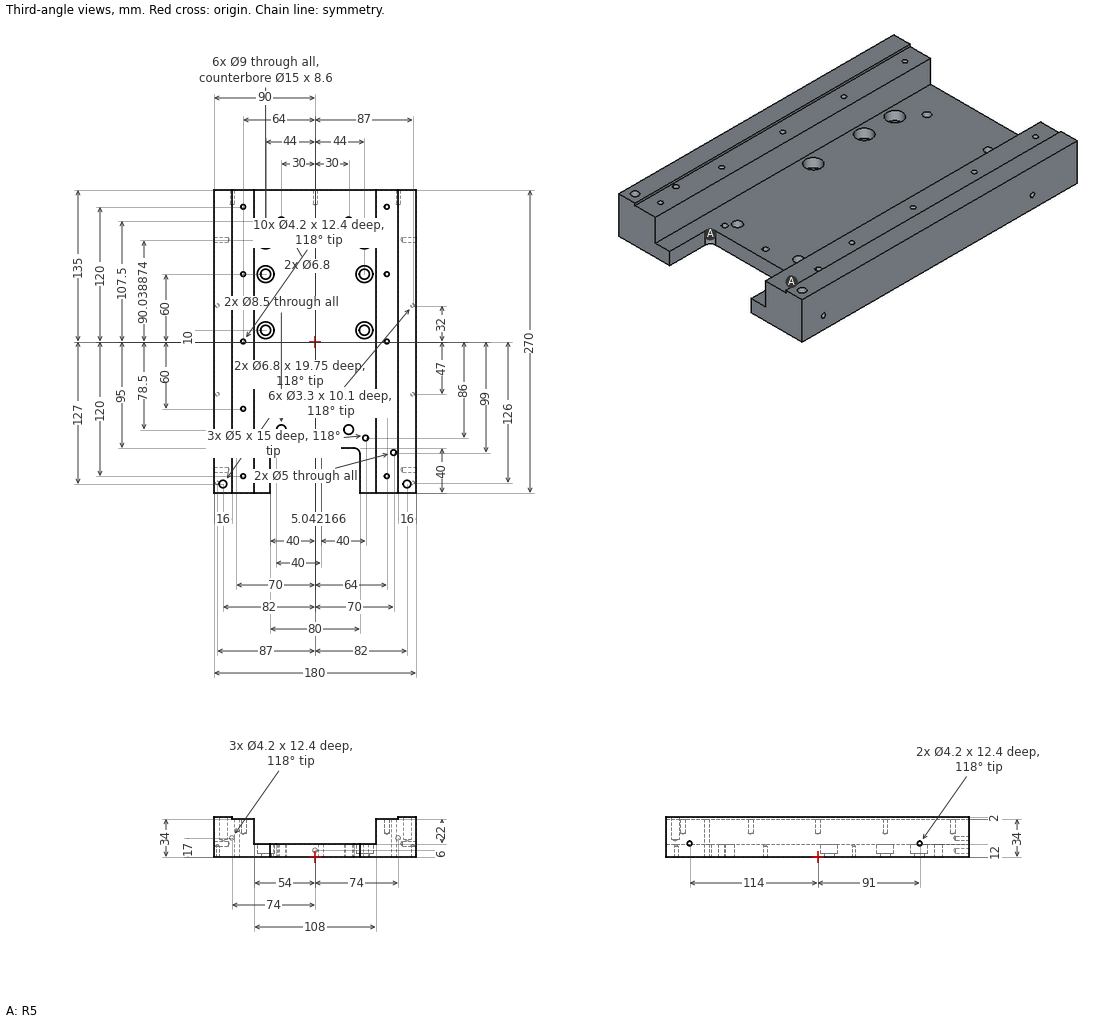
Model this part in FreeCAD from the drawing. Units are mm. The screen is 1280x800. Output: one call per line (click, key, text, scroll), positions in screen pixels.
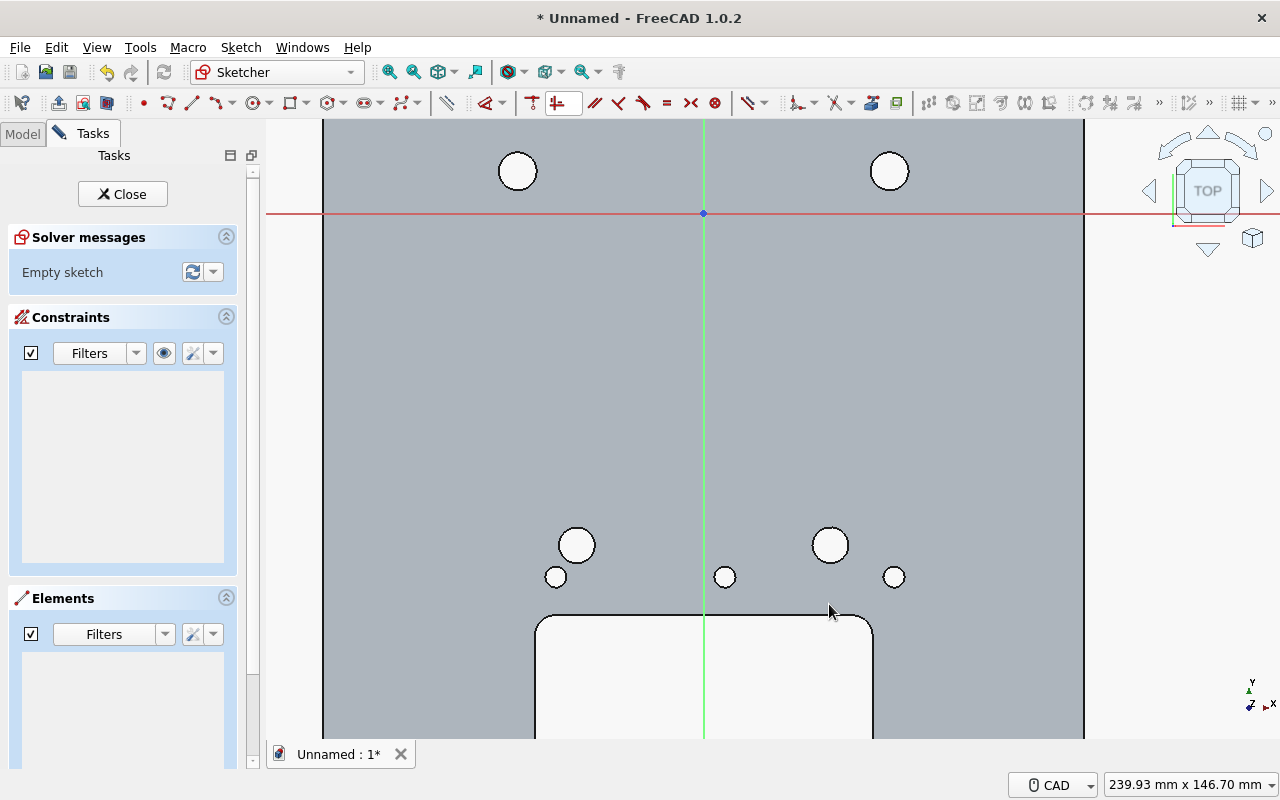
key(g)
key(c)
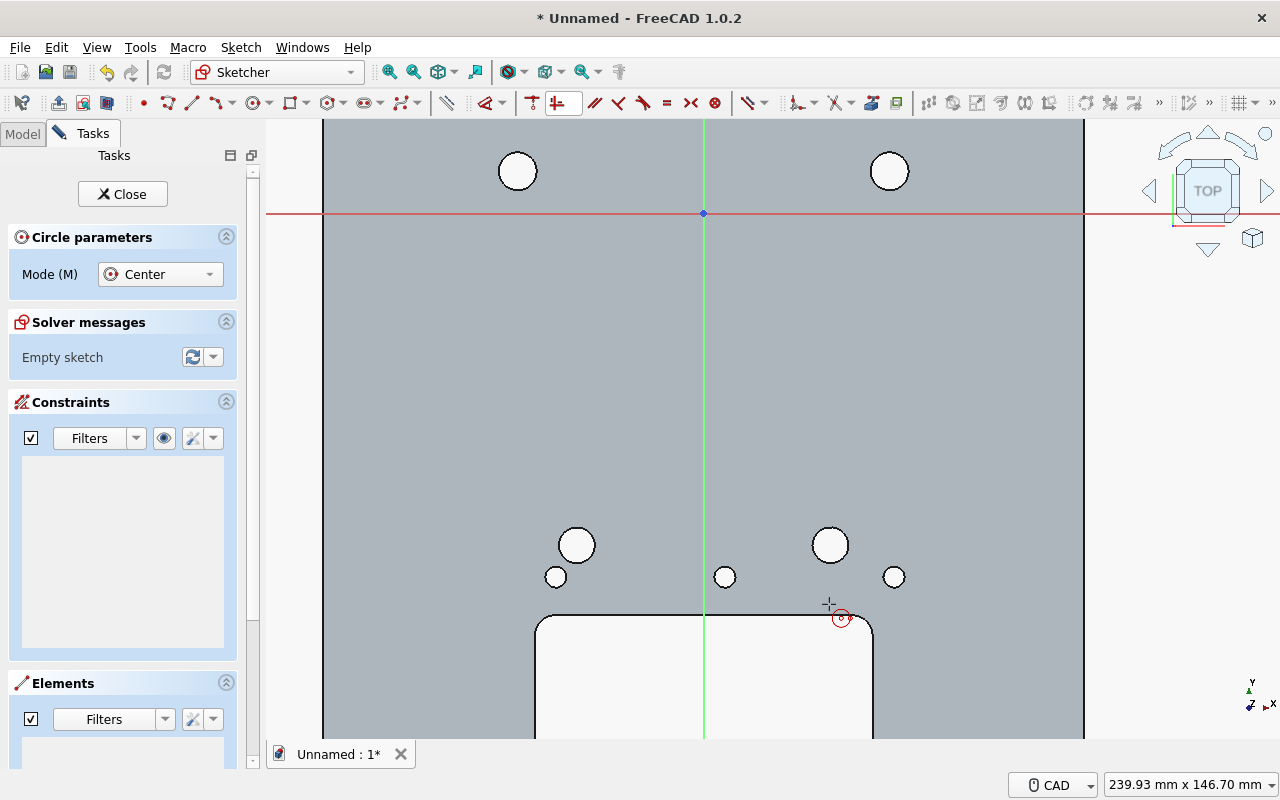
scroll(1000, 632, up, 4)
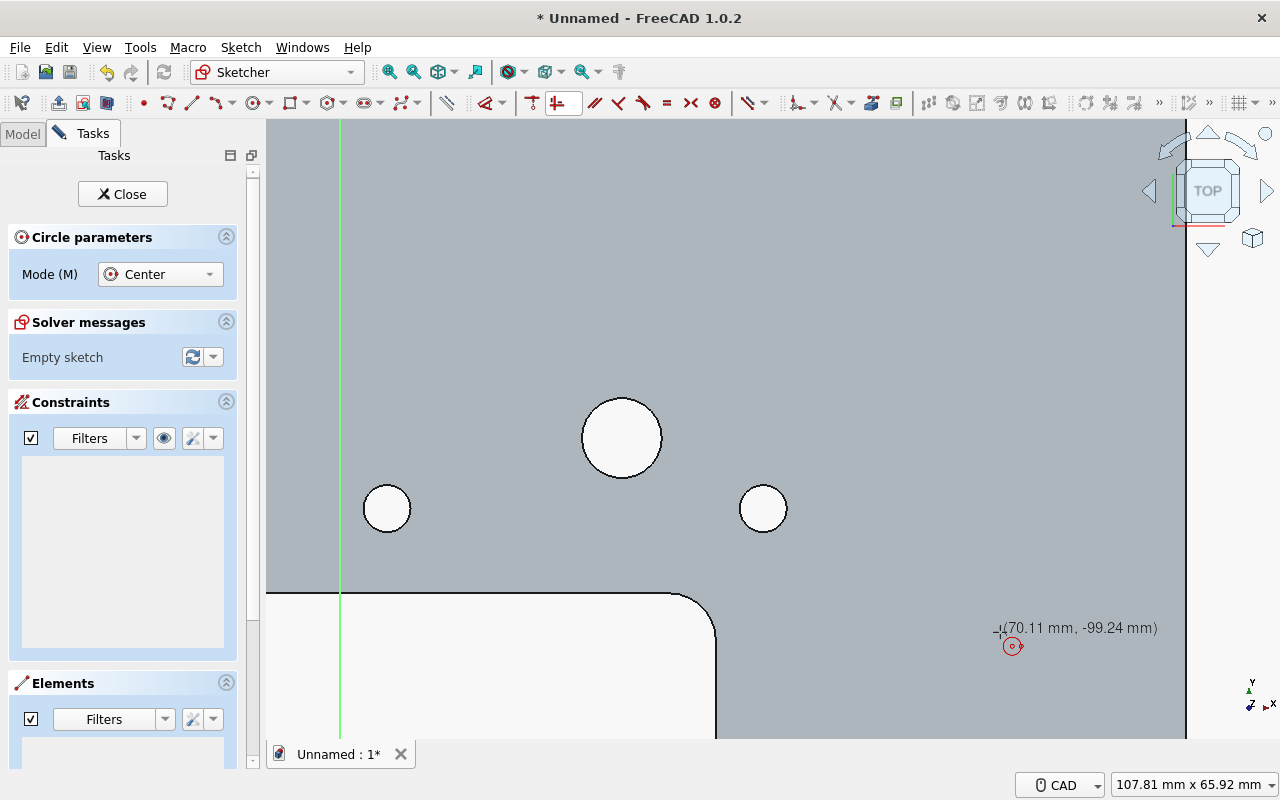
click(998, 631)
move(1015, 614)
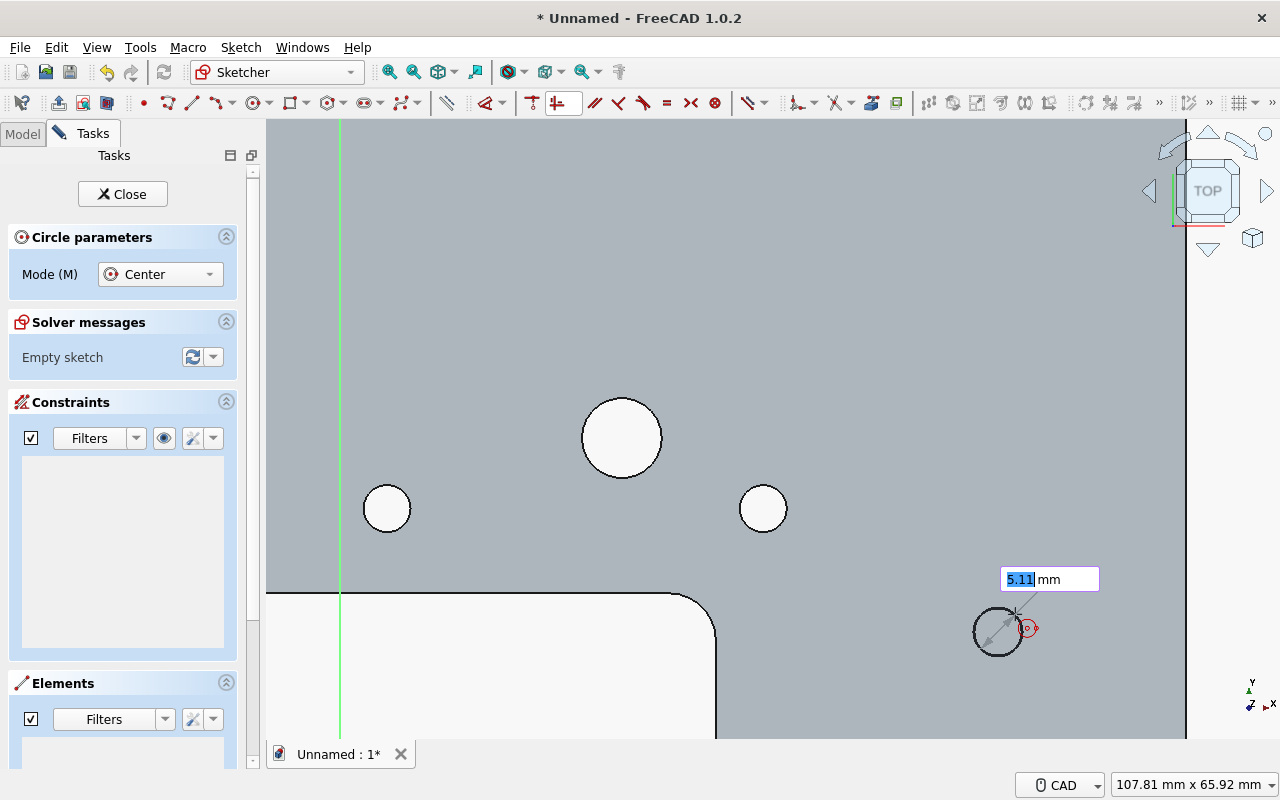
text(5)
key(Return)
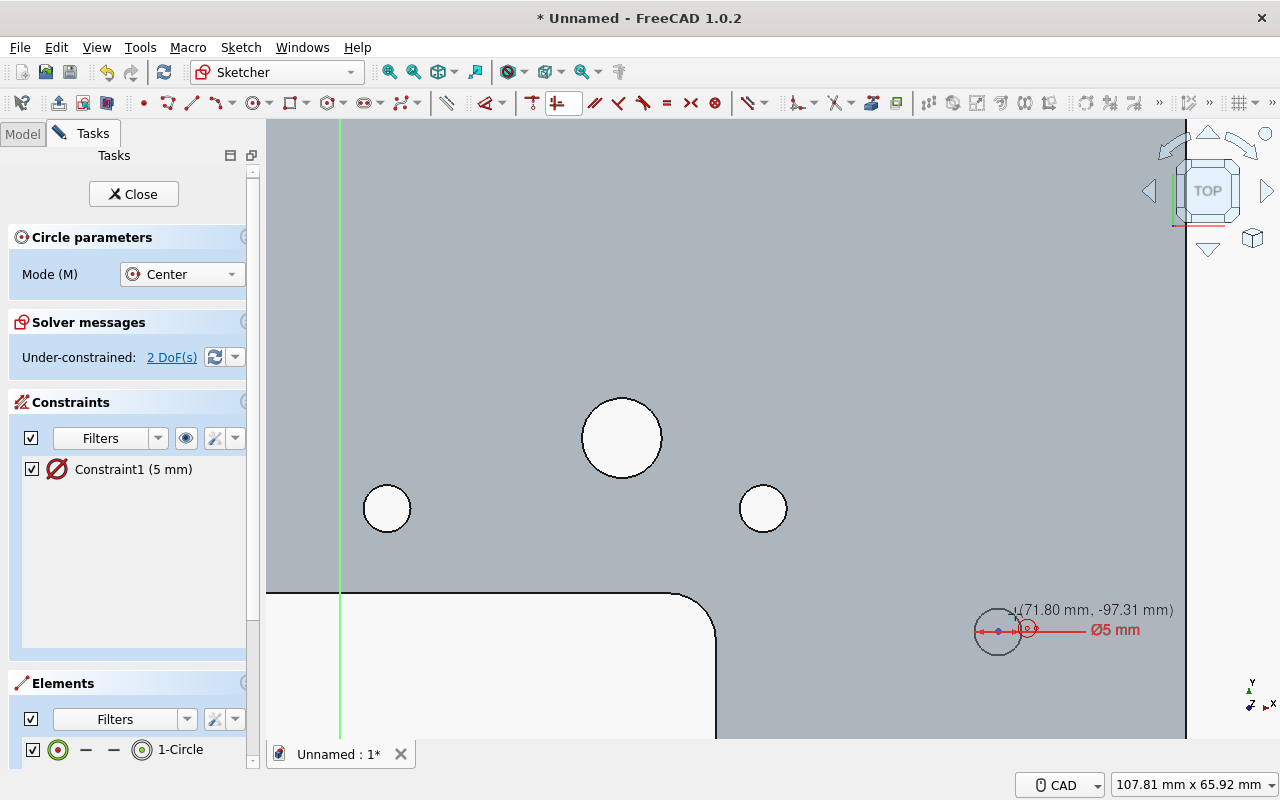
scroll(1002, 635, down, 4)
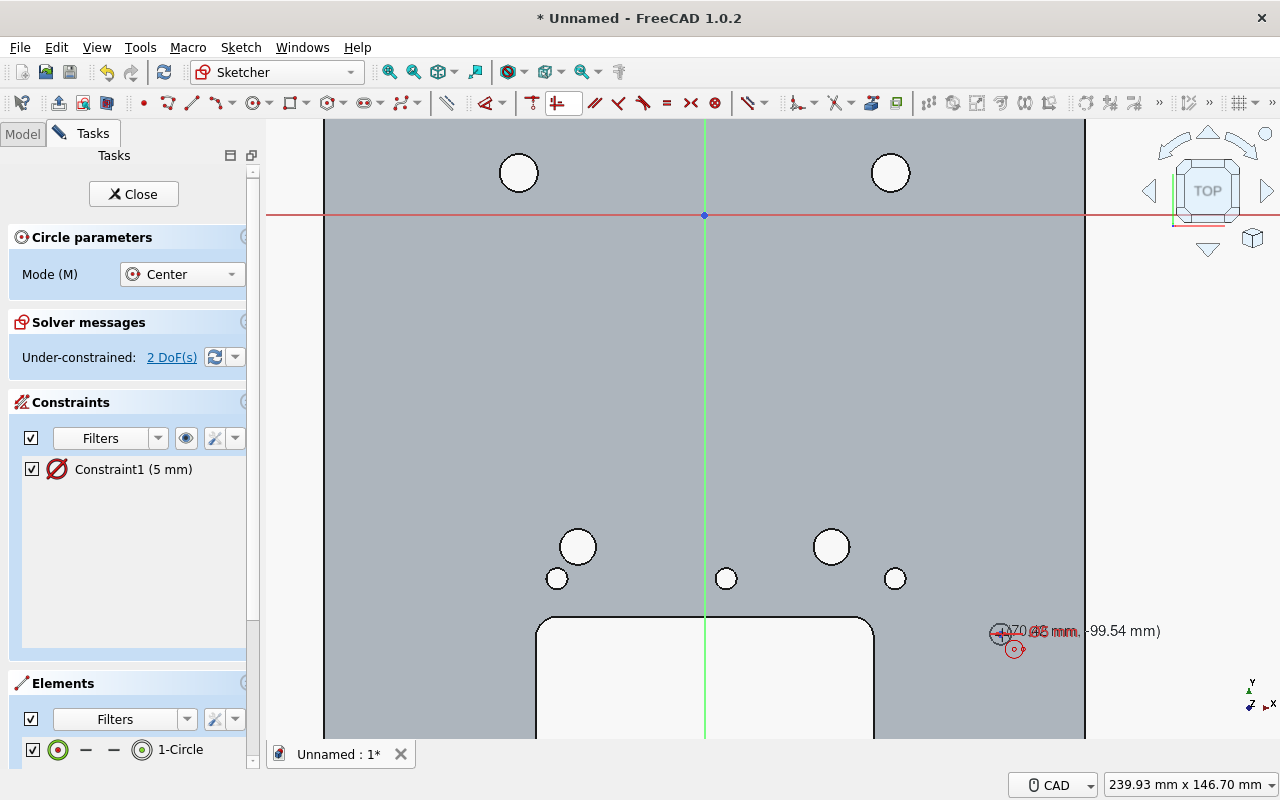
scroll(409, 634, up, 4)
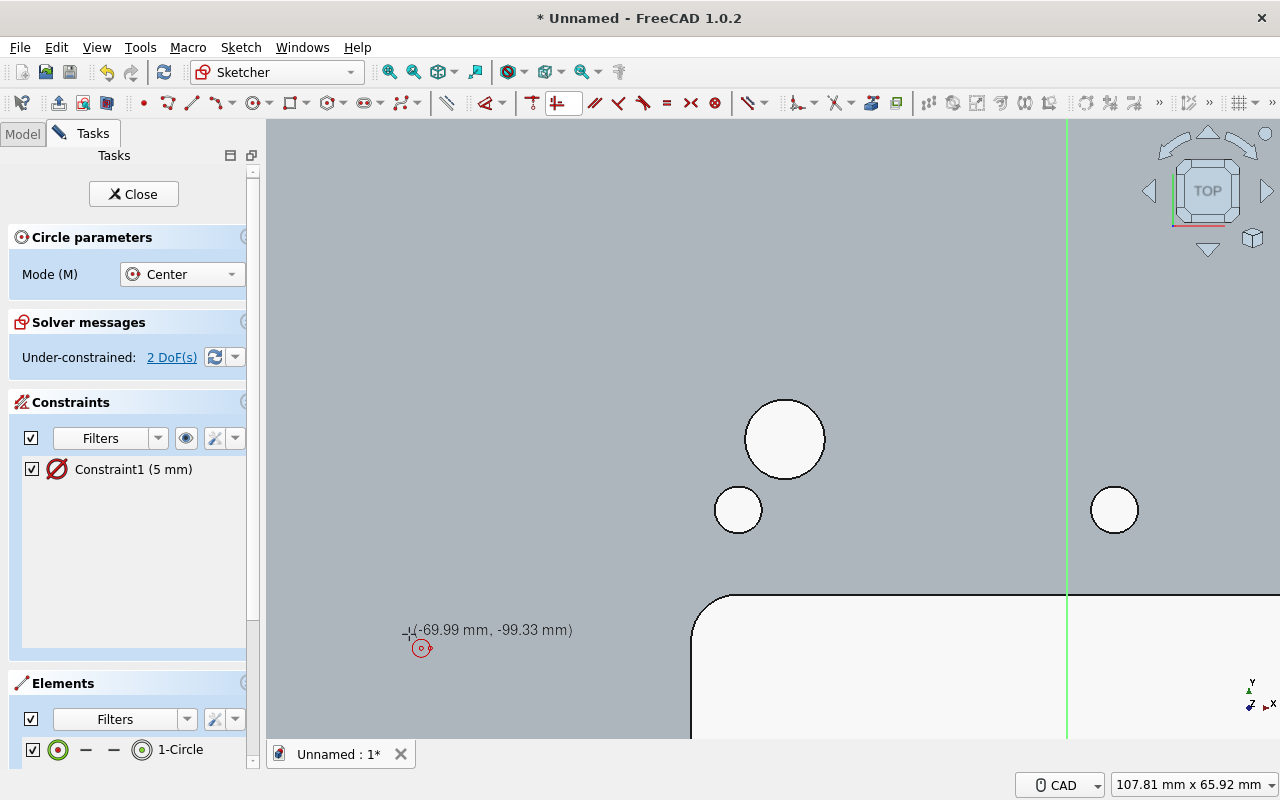
click(409, 632)
move(425, 616)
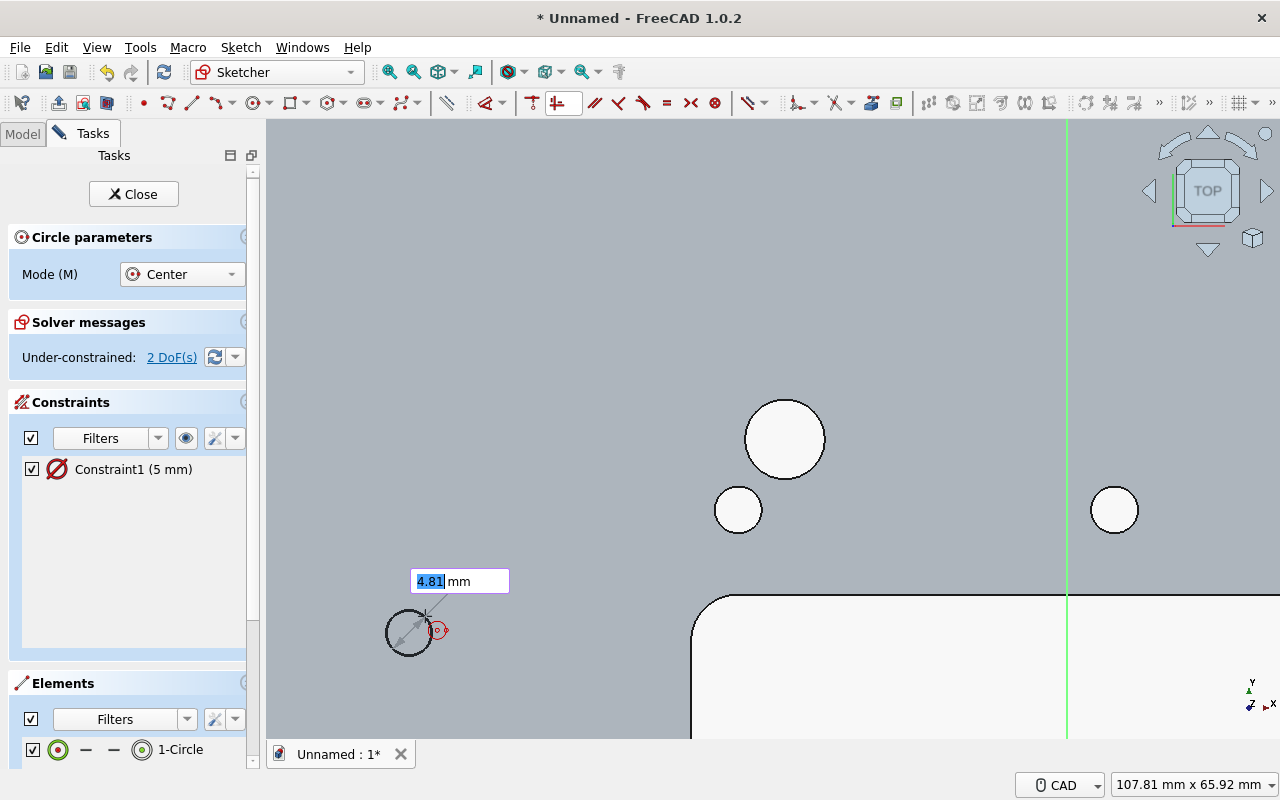
text(5)
key(Return)
key(Escape)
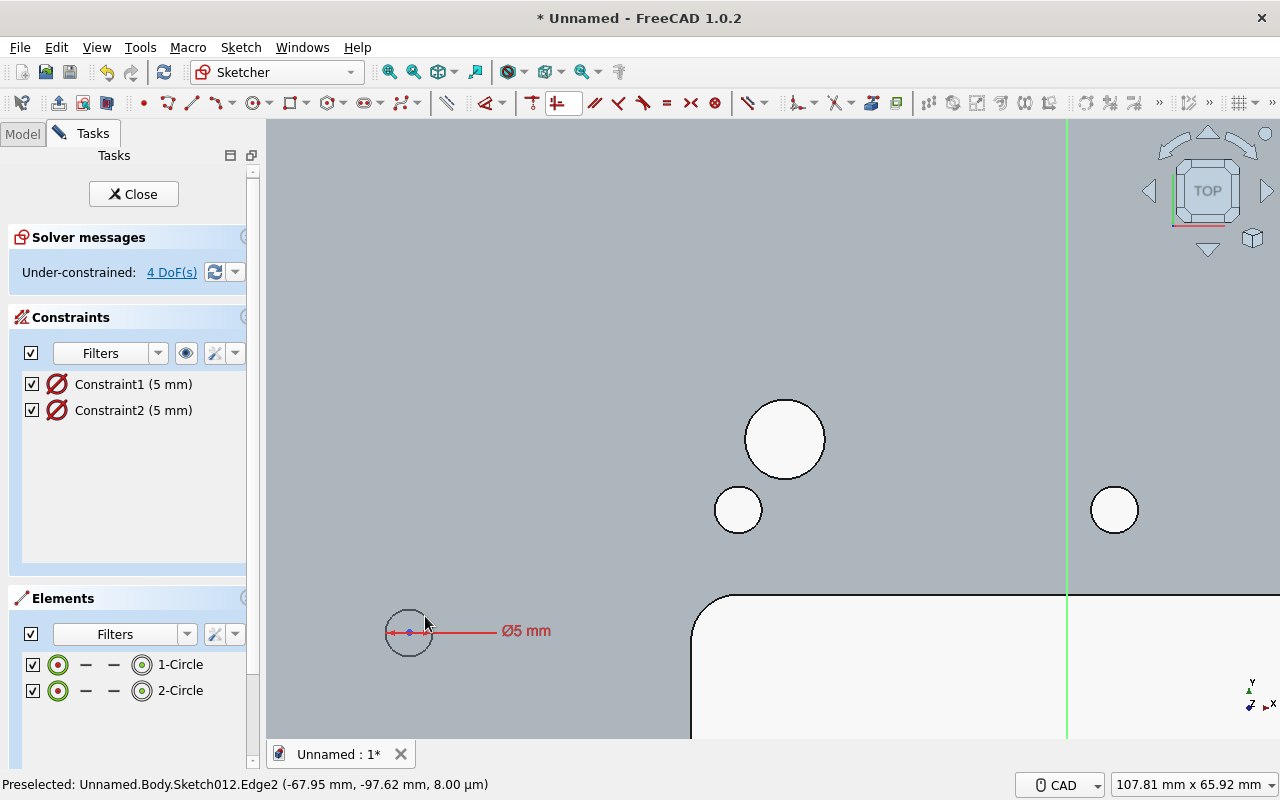
scroll(409, 634, down, 4)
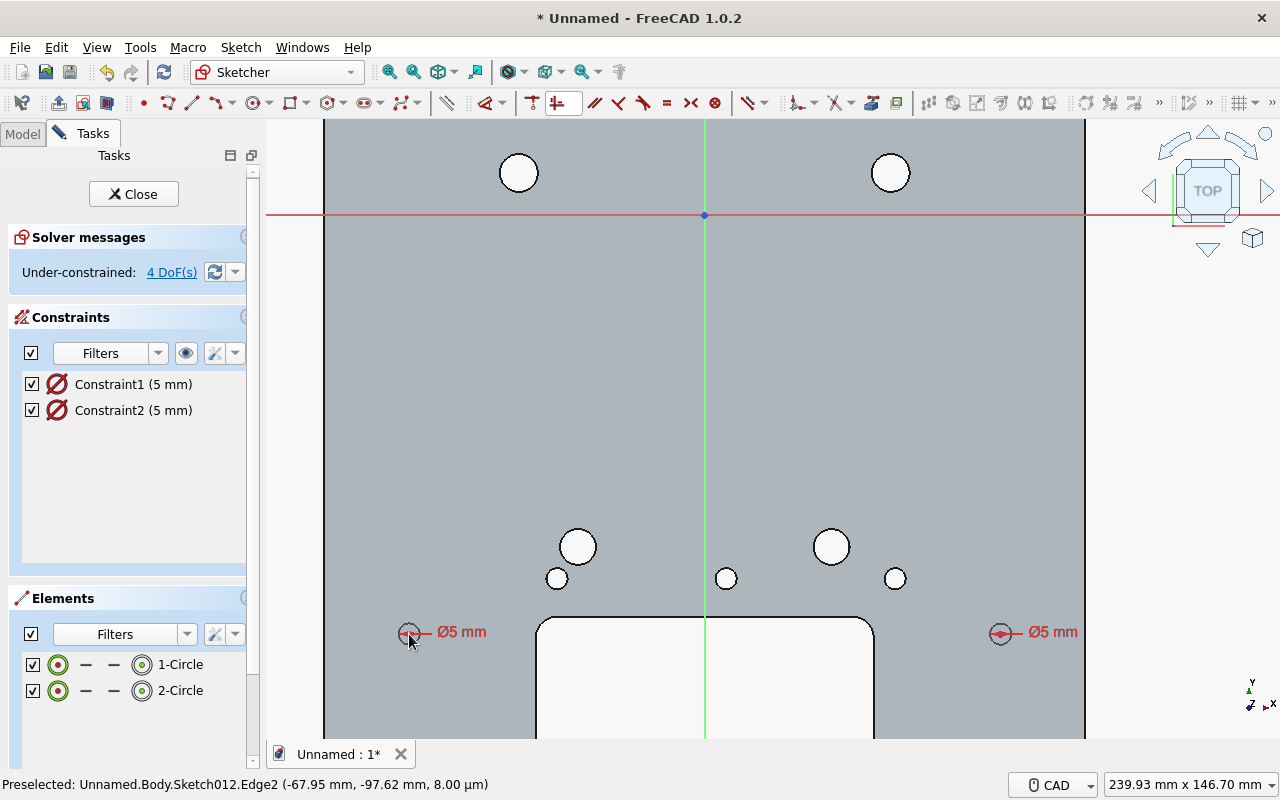
click(1001, 634)